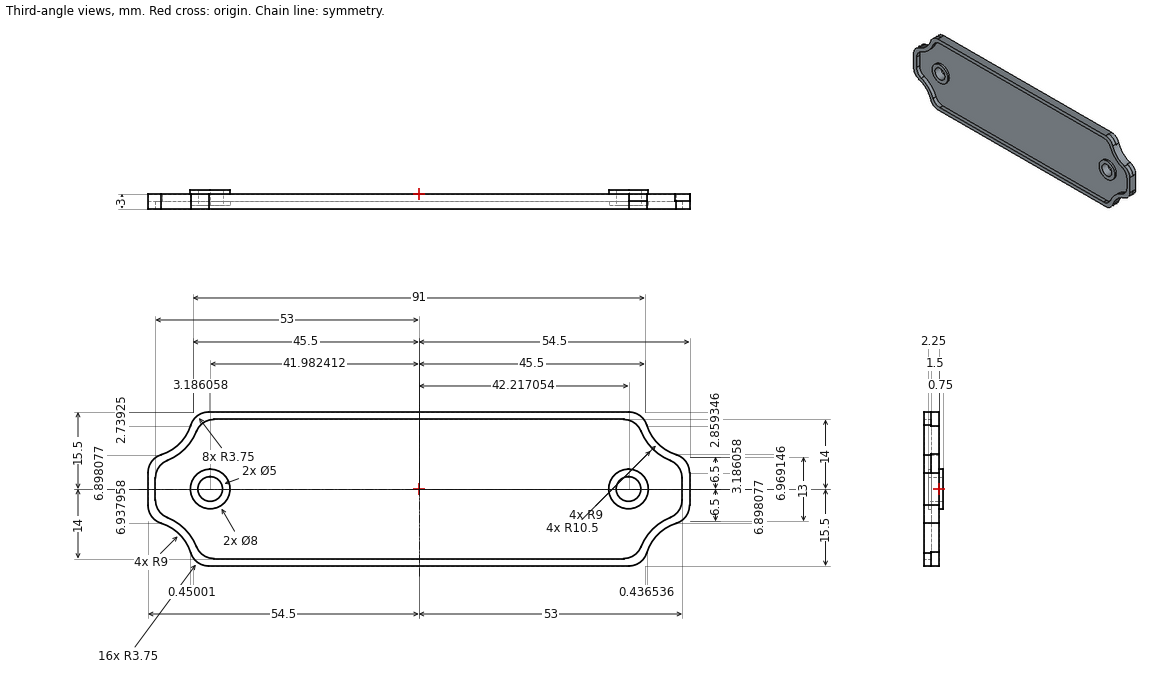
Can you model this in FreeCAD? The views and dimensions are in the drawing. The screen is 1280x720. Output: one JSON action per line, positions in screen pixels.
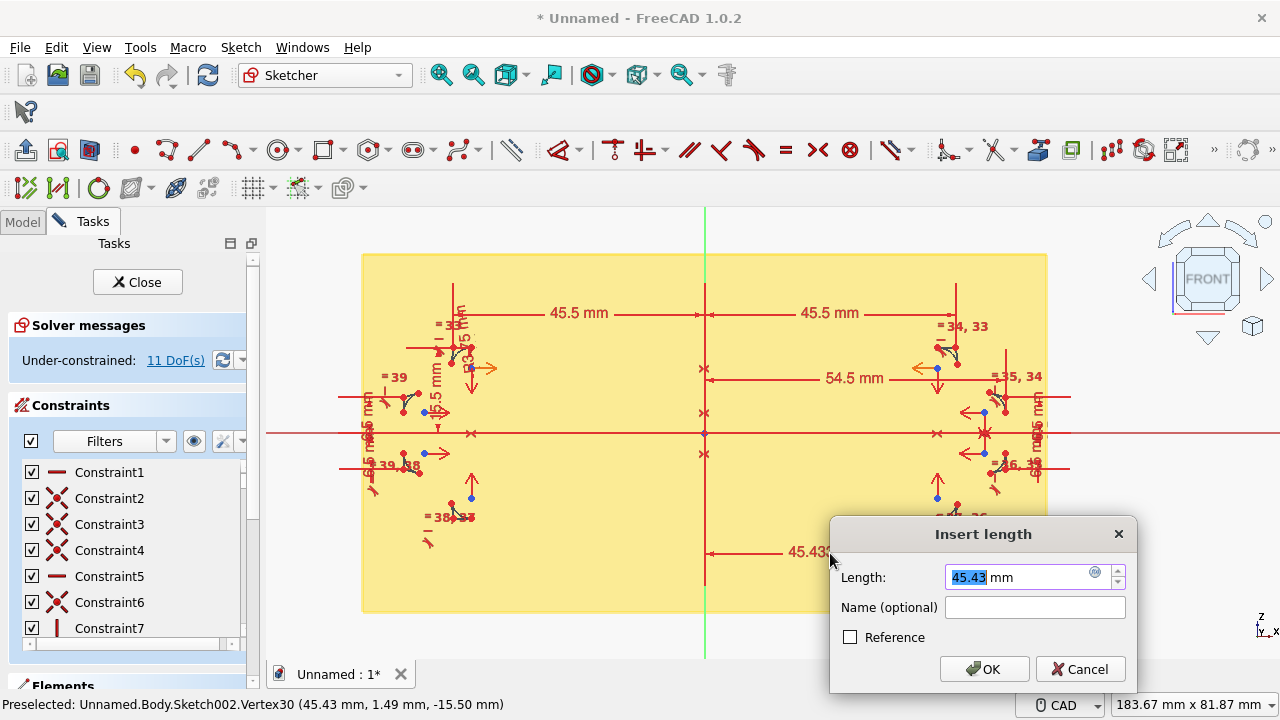
{"action": "type", "text": "45.5"}
{"action": "key", "text": "Return"}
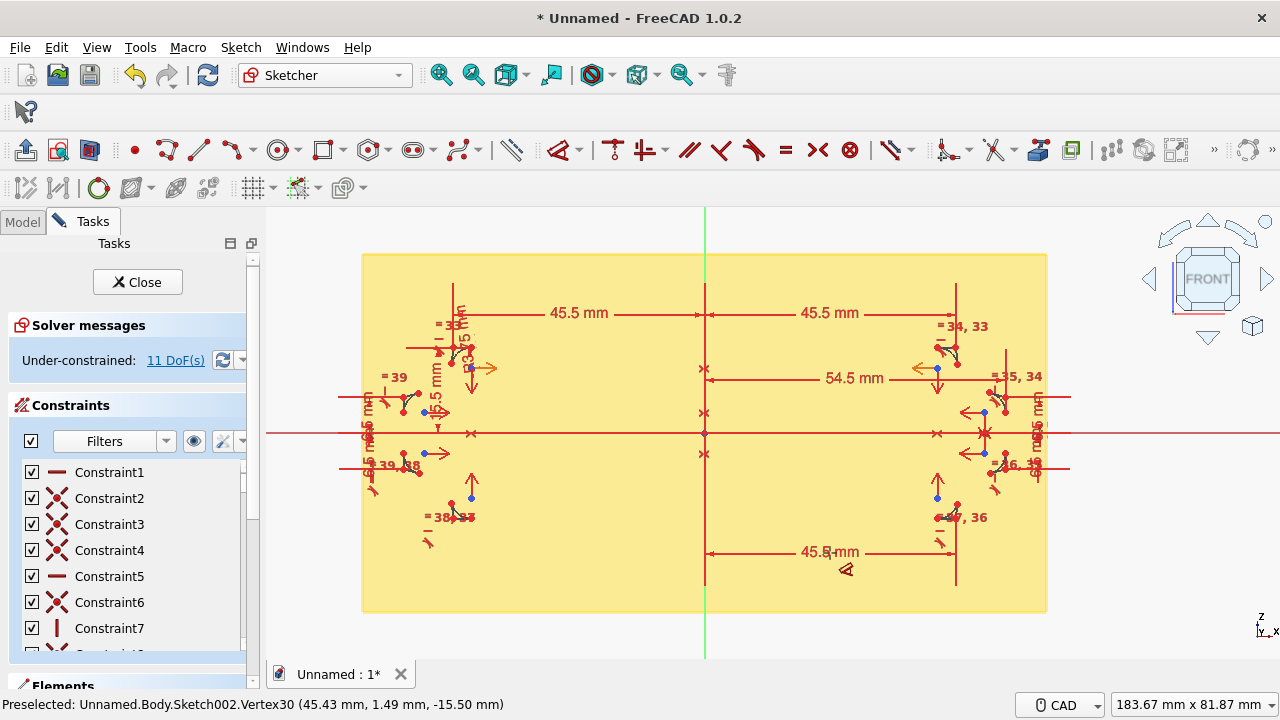
{"action": "left_click", "coordinate": [454, 519]}
{"action": "left_click", "coordinate": [579, 553]}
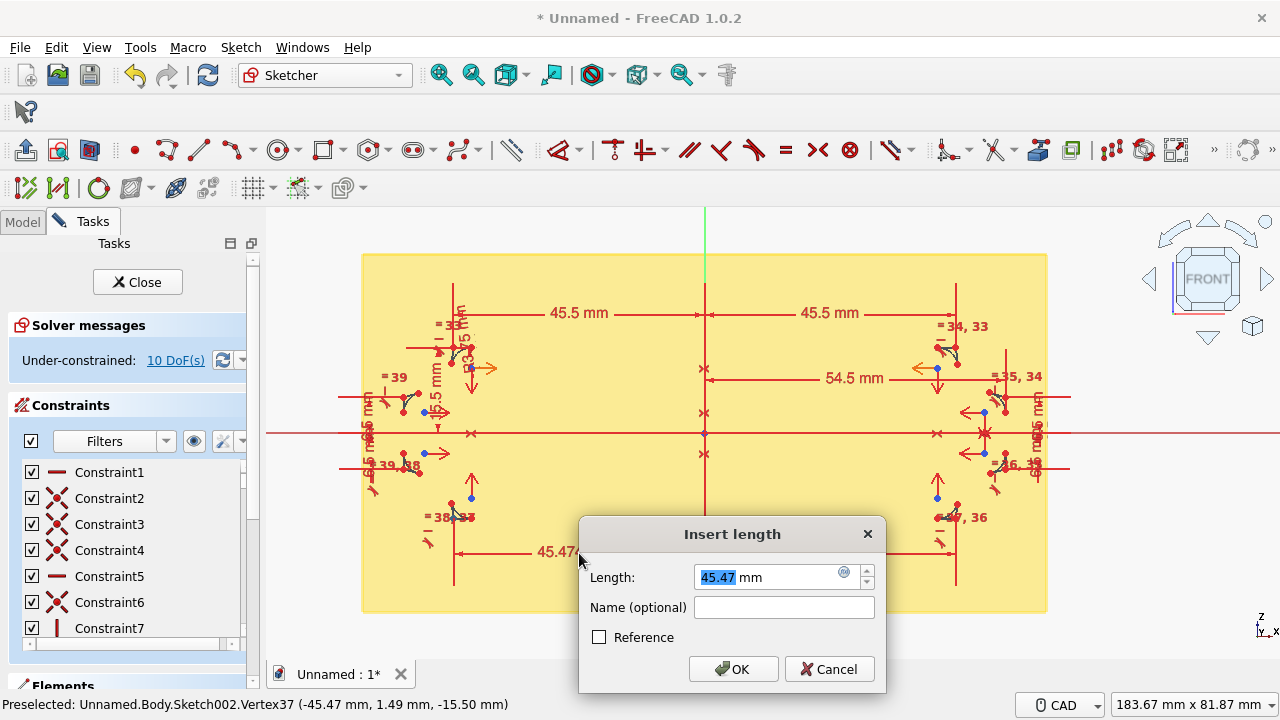
{"action": "type", "text": "45.5"}
{"action": "key", "text": "Return"}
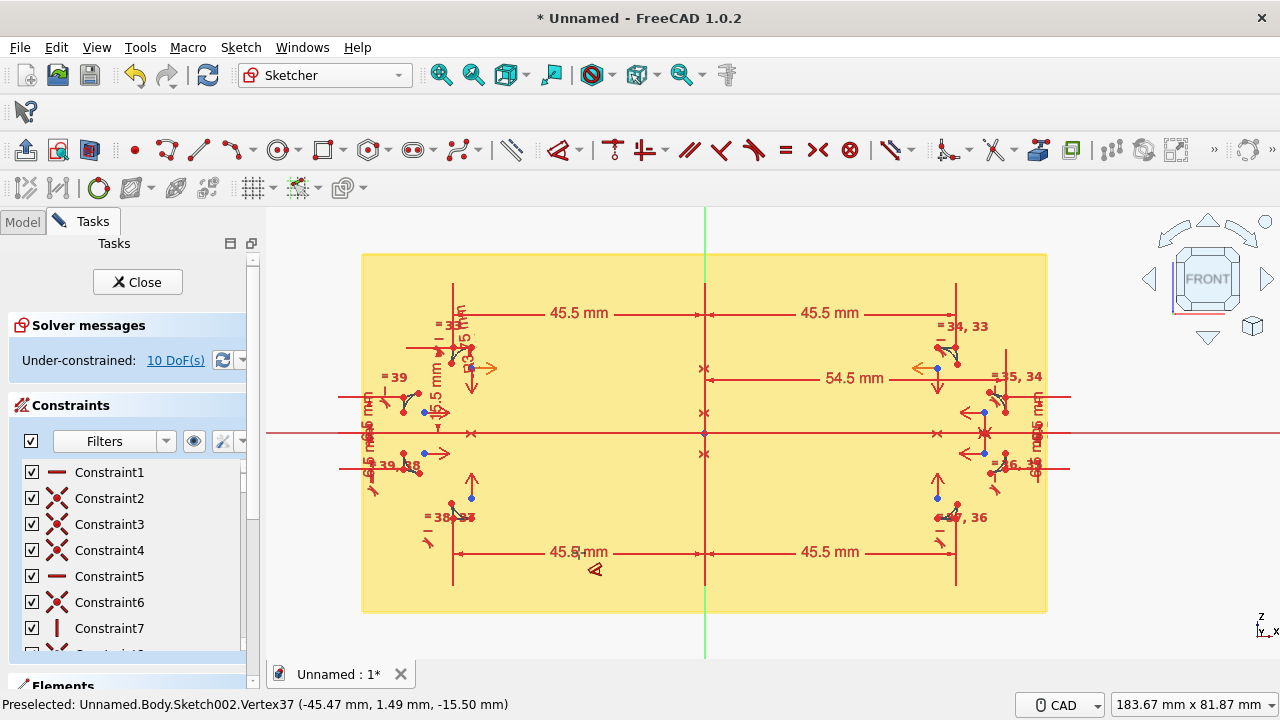
{"action": "scroll", "coordinate": [457, 348], "scroll_direction": "up", "scroll_amount": 7}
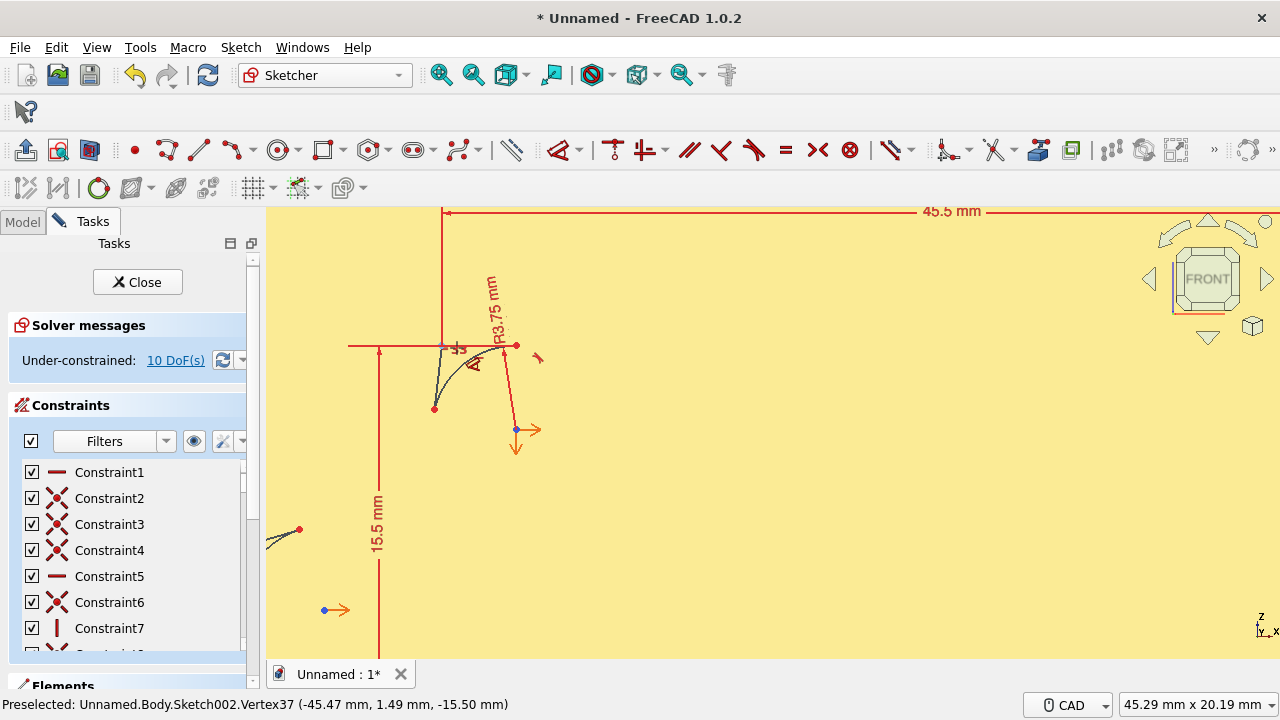
{"action": "left_click", "coordinate": [457, 346]}
{"action": "left_click", "coordinate": [479, 380]}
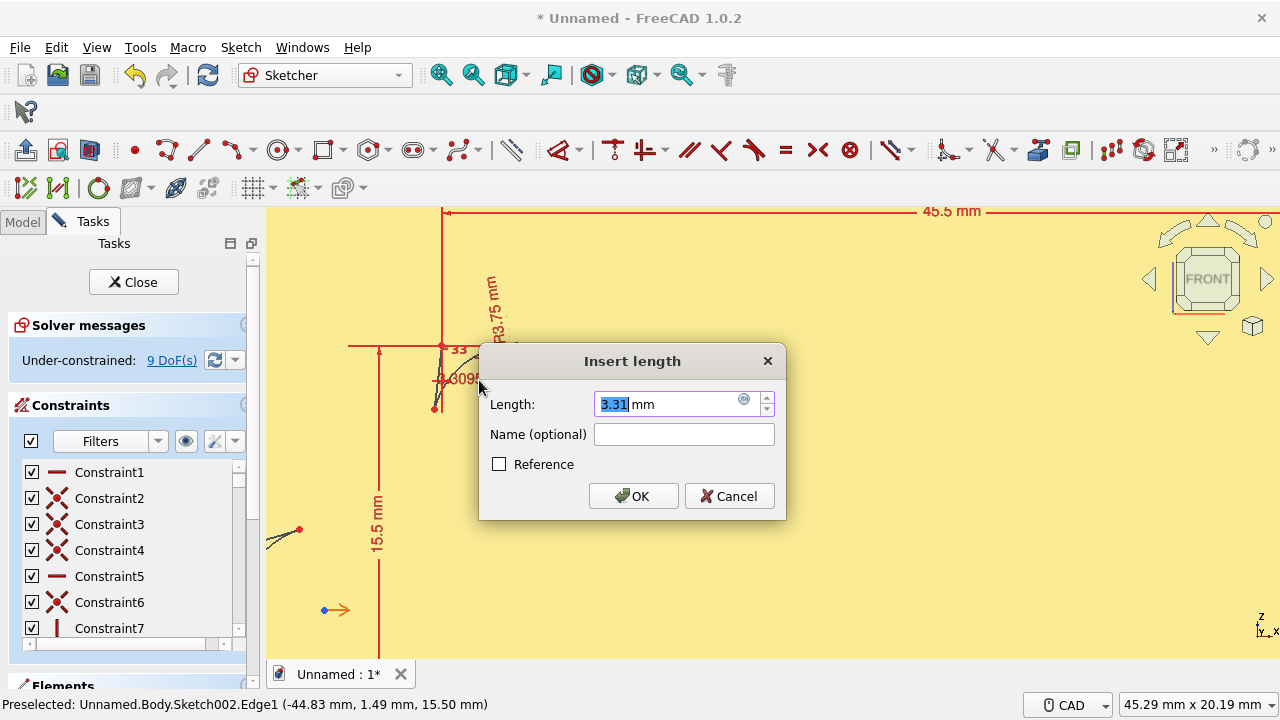
{"action": "type", "text": "3.186058"}
{"action": "key", "text": "Return"}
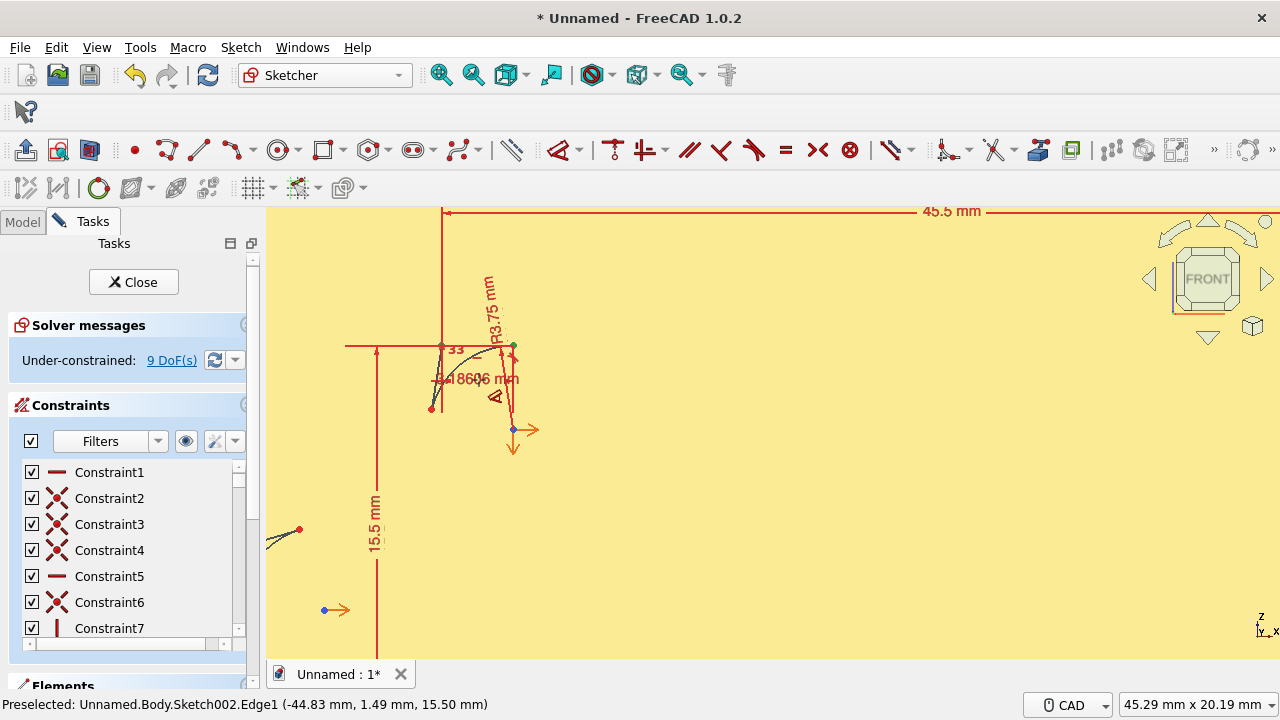
{"action": "scroll", "coordinate": [457, 348], "scroll_direction": "down", "scroll_amount": 7}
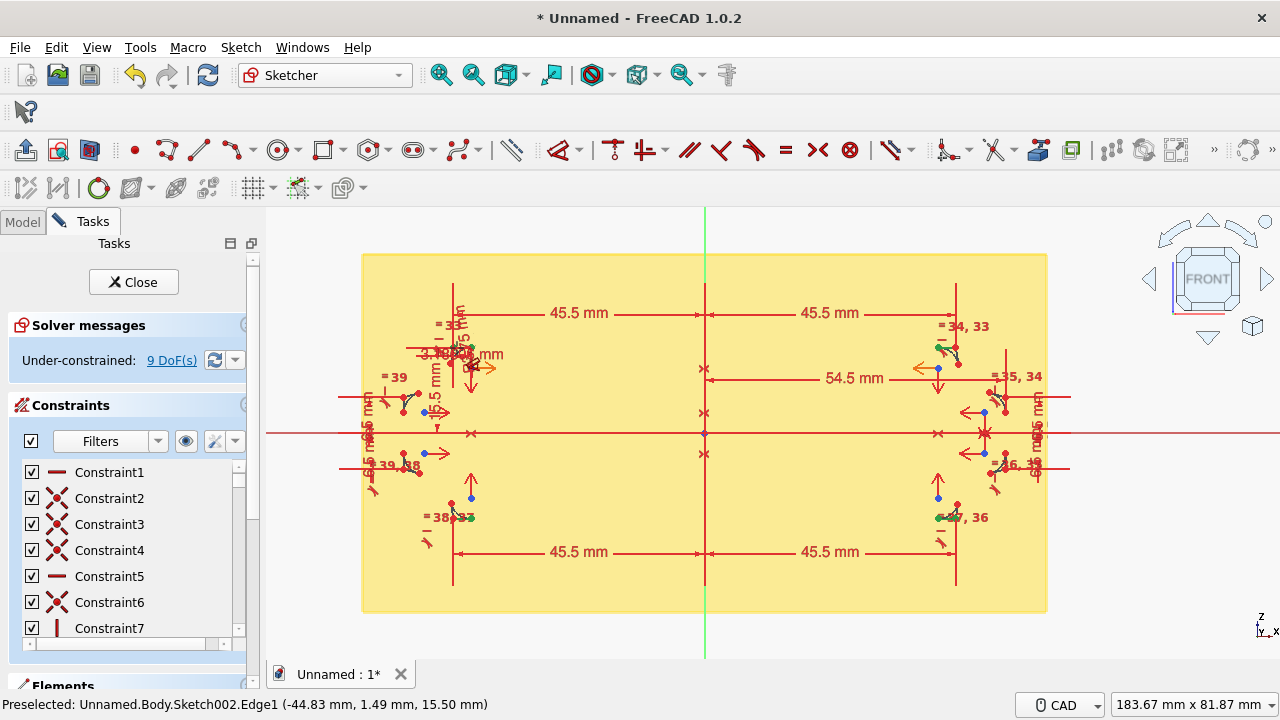
{"action": "scroll", "coordinate": [1006, 402], "scroll_direction": "up", "scroll_amount": 9}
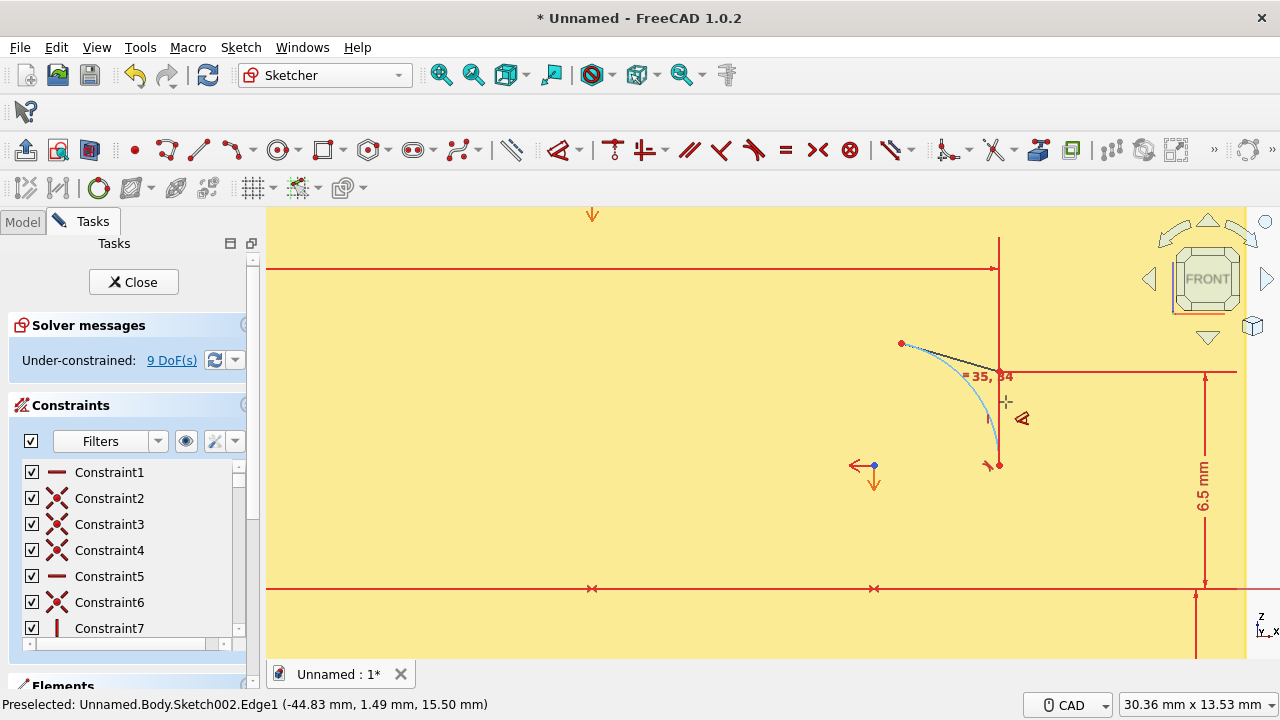
{"action": "left_click", "coordinate": [999, 400]}
{"action": "left_click", "coordinate": [1033, 419]}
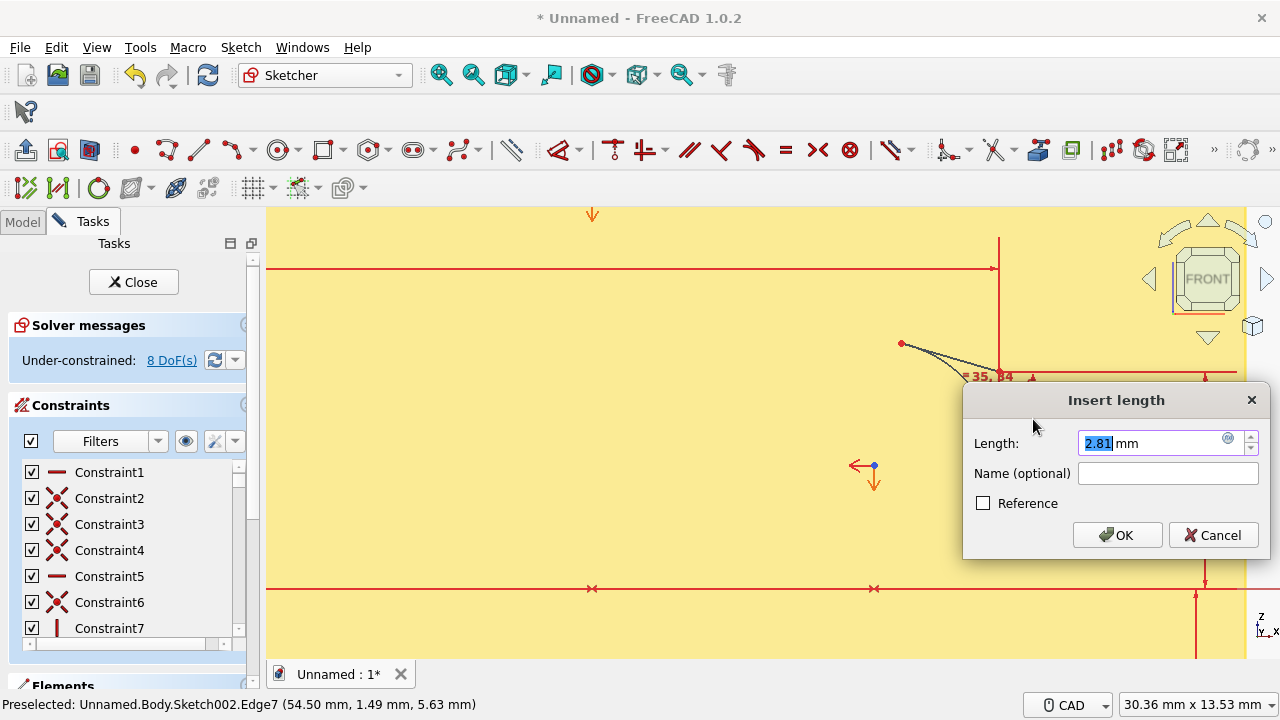
{"action": "type", "text": "3.186058"}
{"action": "key", "text": "Return"}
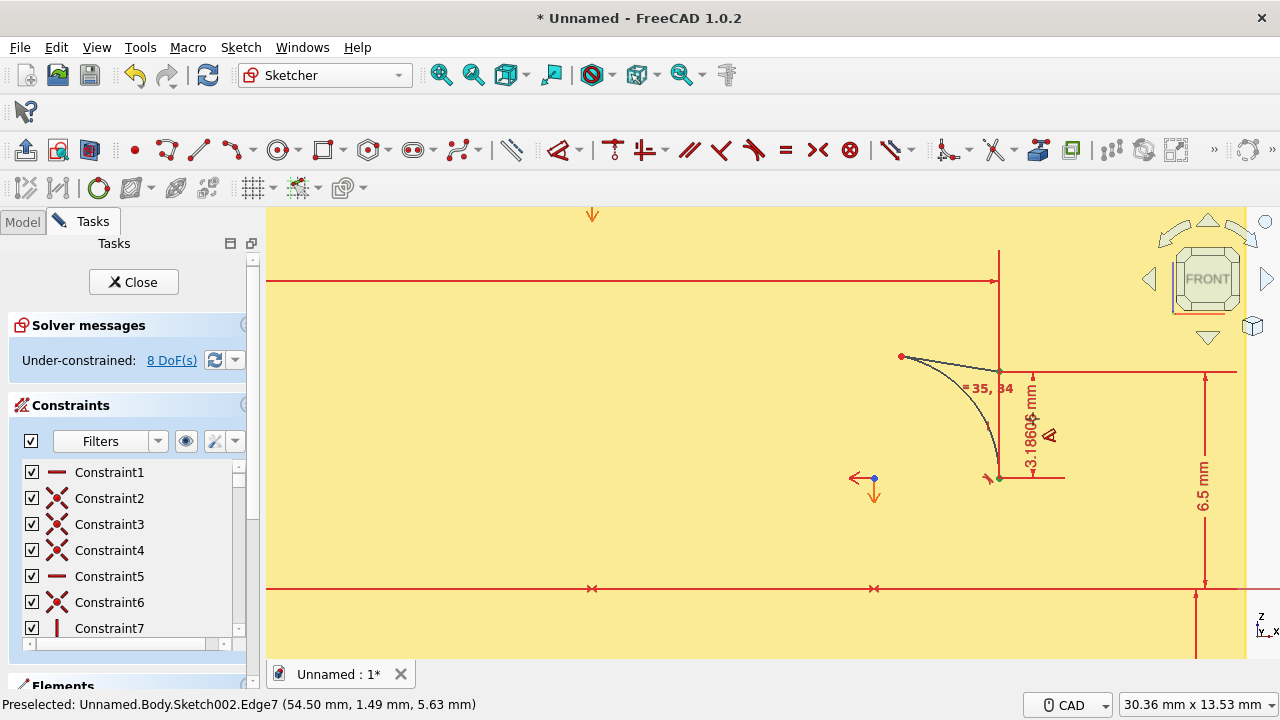
{"action": "scroll", "coordinate": [1007, 402], "scroll_direction": "down", "scroll_amount": 9}